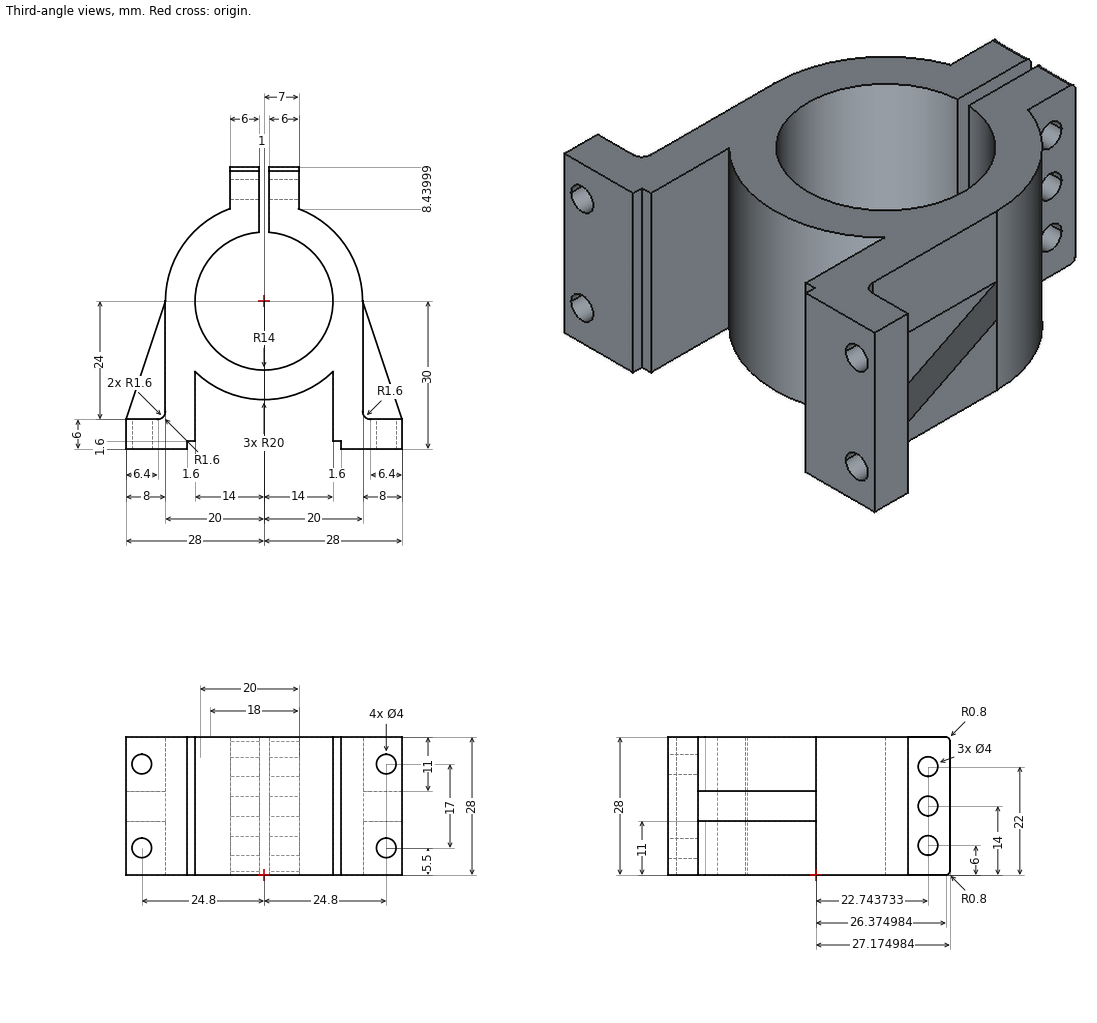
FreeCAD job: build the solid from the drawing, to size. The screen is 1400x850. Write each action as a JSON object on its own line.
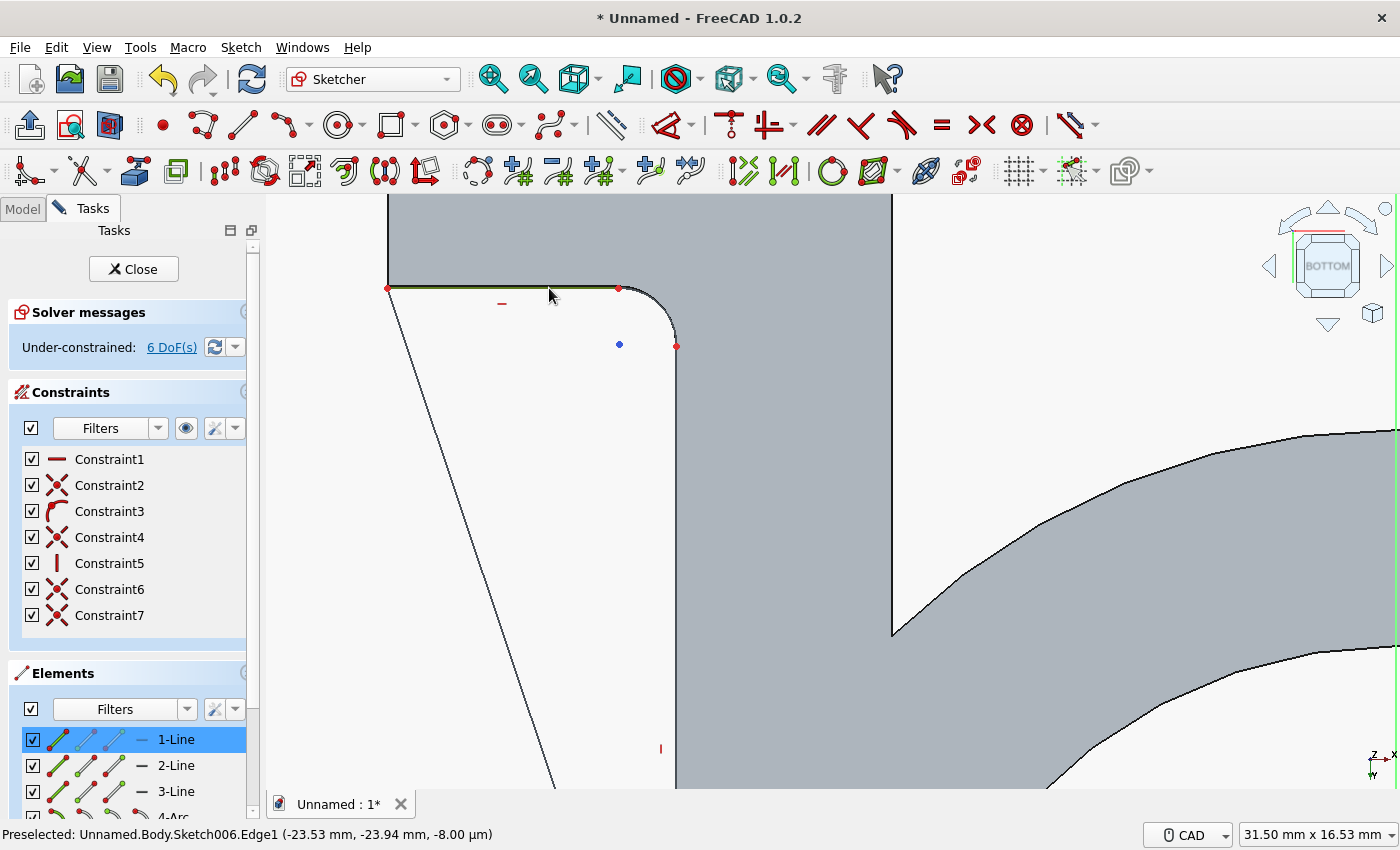
{"action": "left_click", "coordinate": [670, 320]}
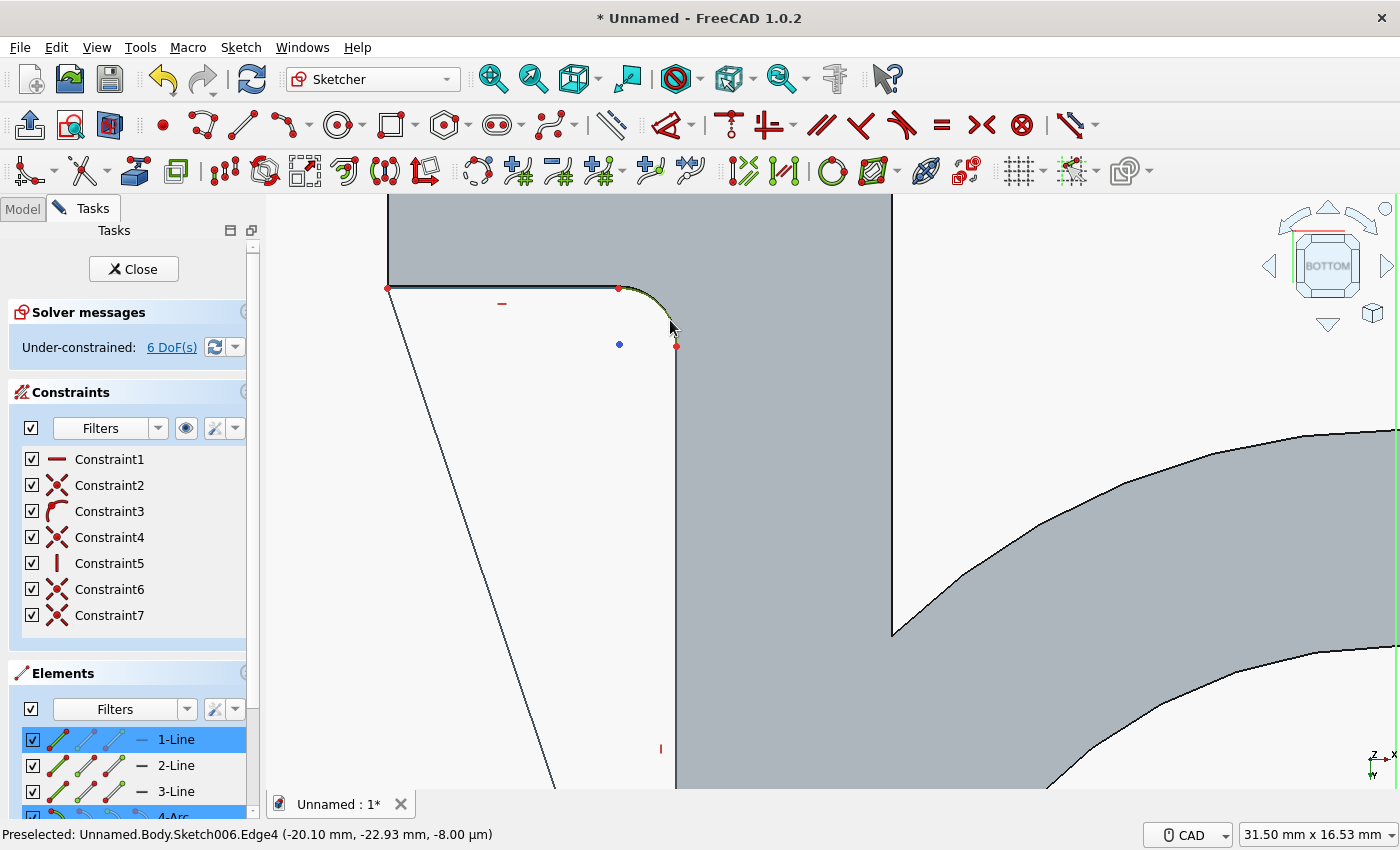
{"action": "left_click", "coordinate": [902, 126]}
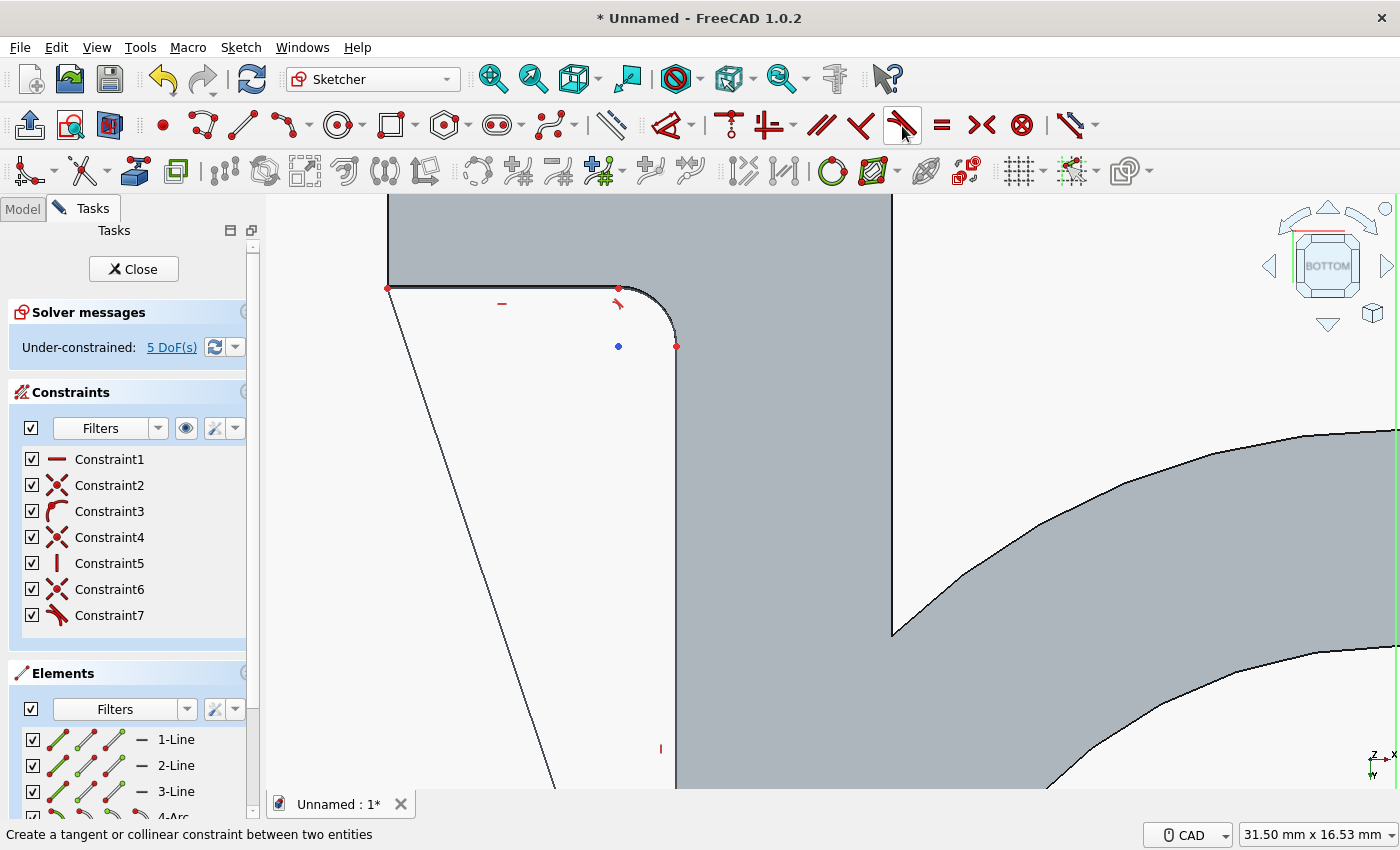
{"action": "left_click", "coordinate": [676, 587]}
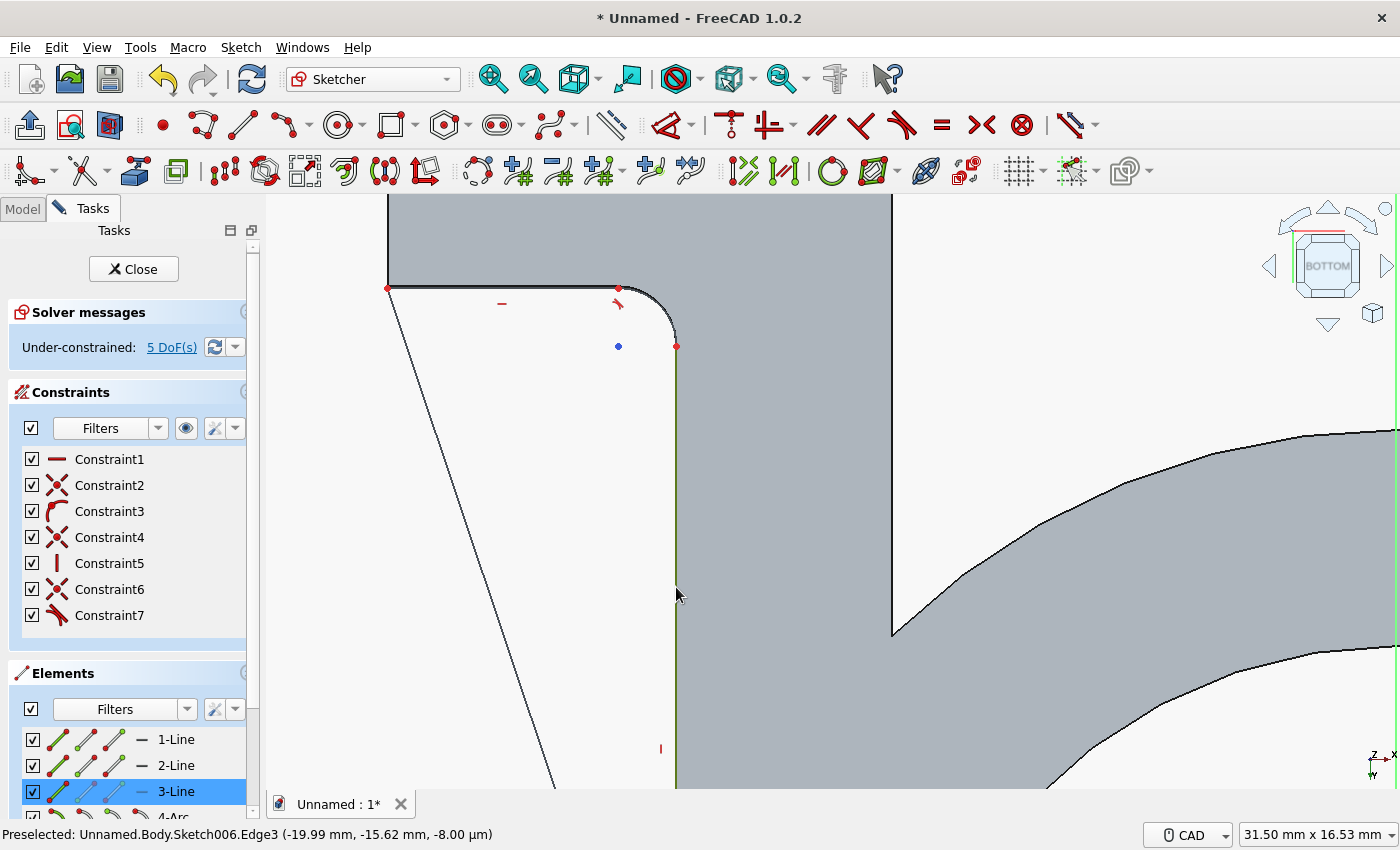
{"action": "left_click", "coordinate": [670, 320]}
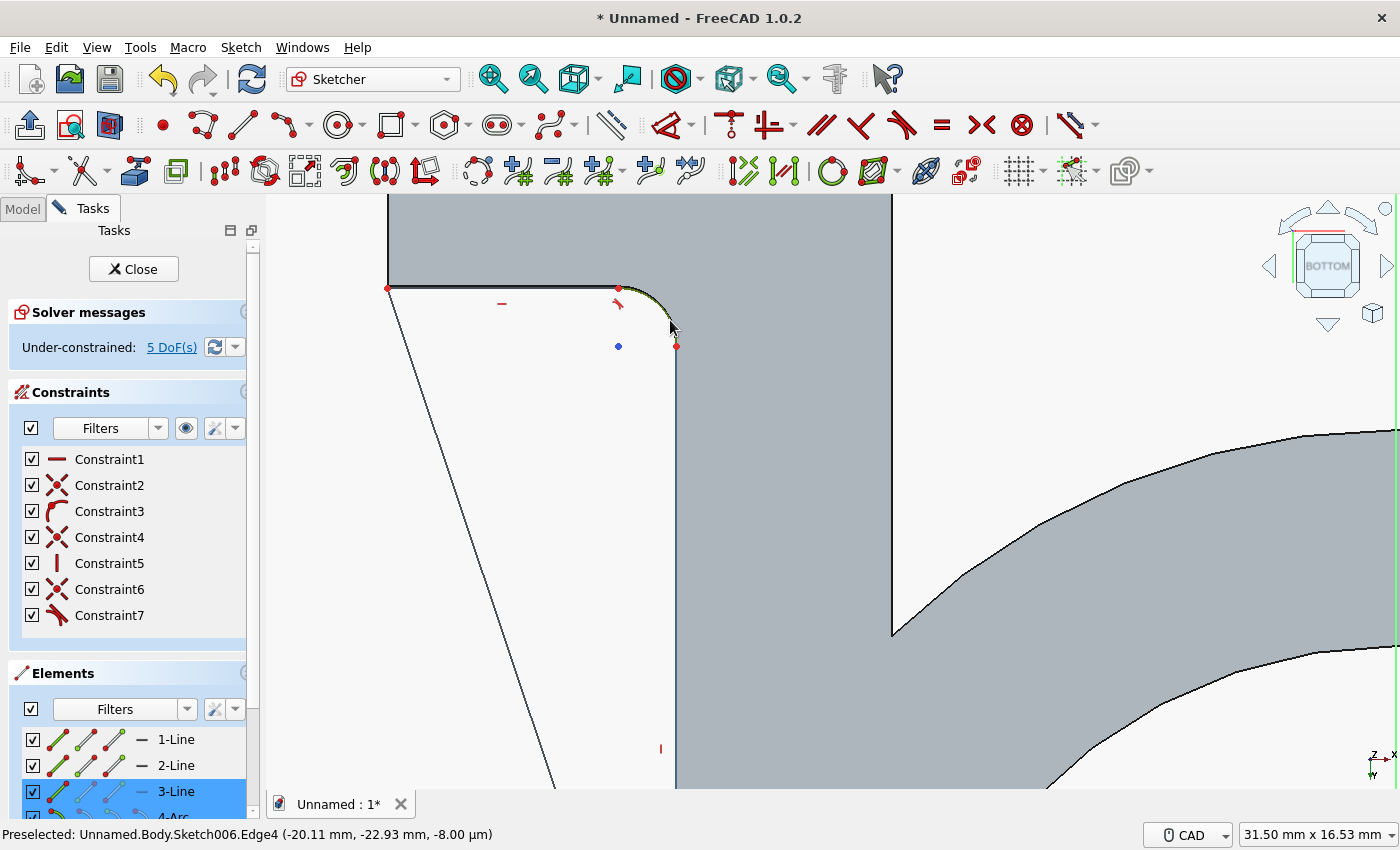
{"action": "left_click", "coordinate": [902, 126]}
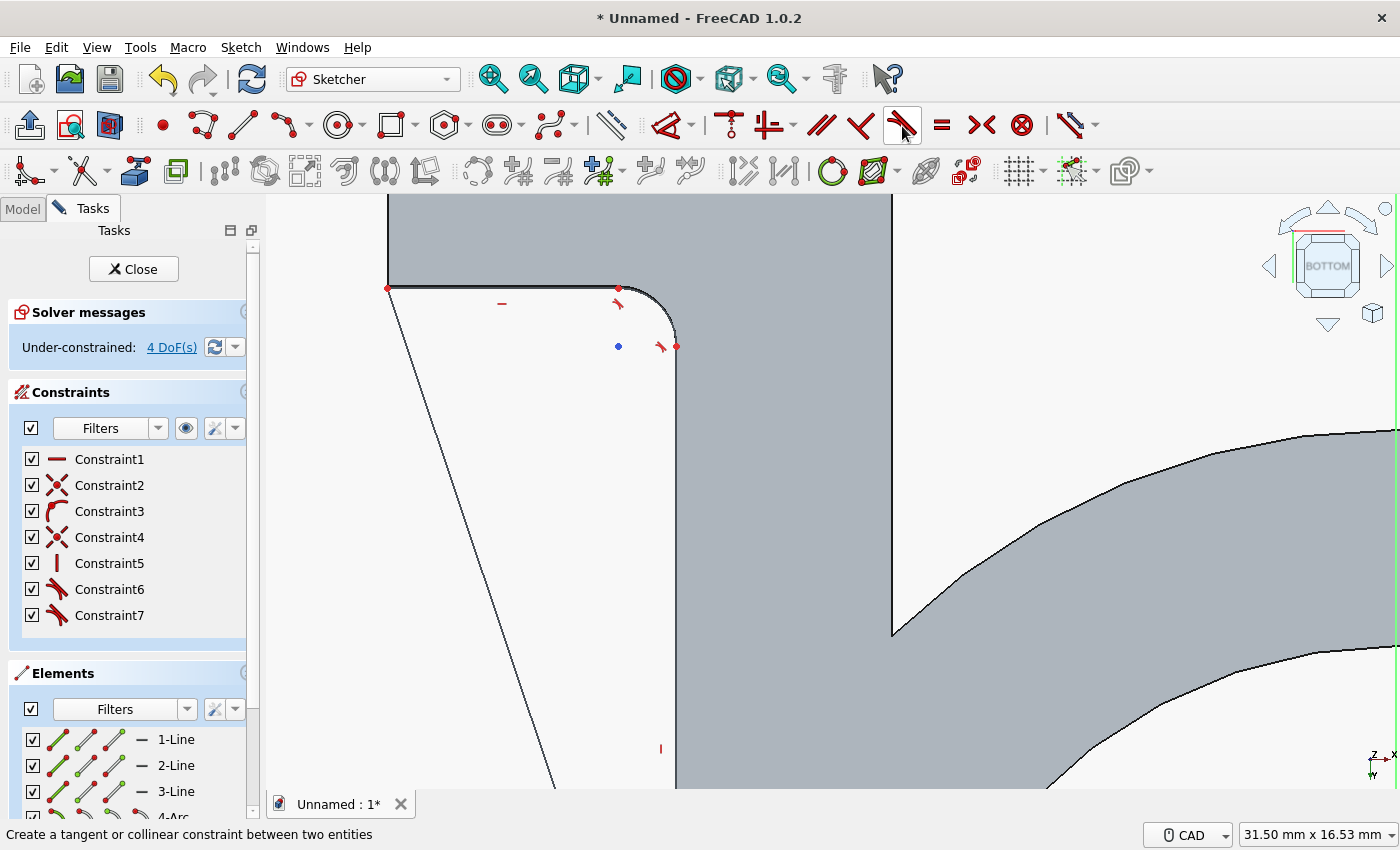
{"action": "left_click", "coordinate": [666, 126]}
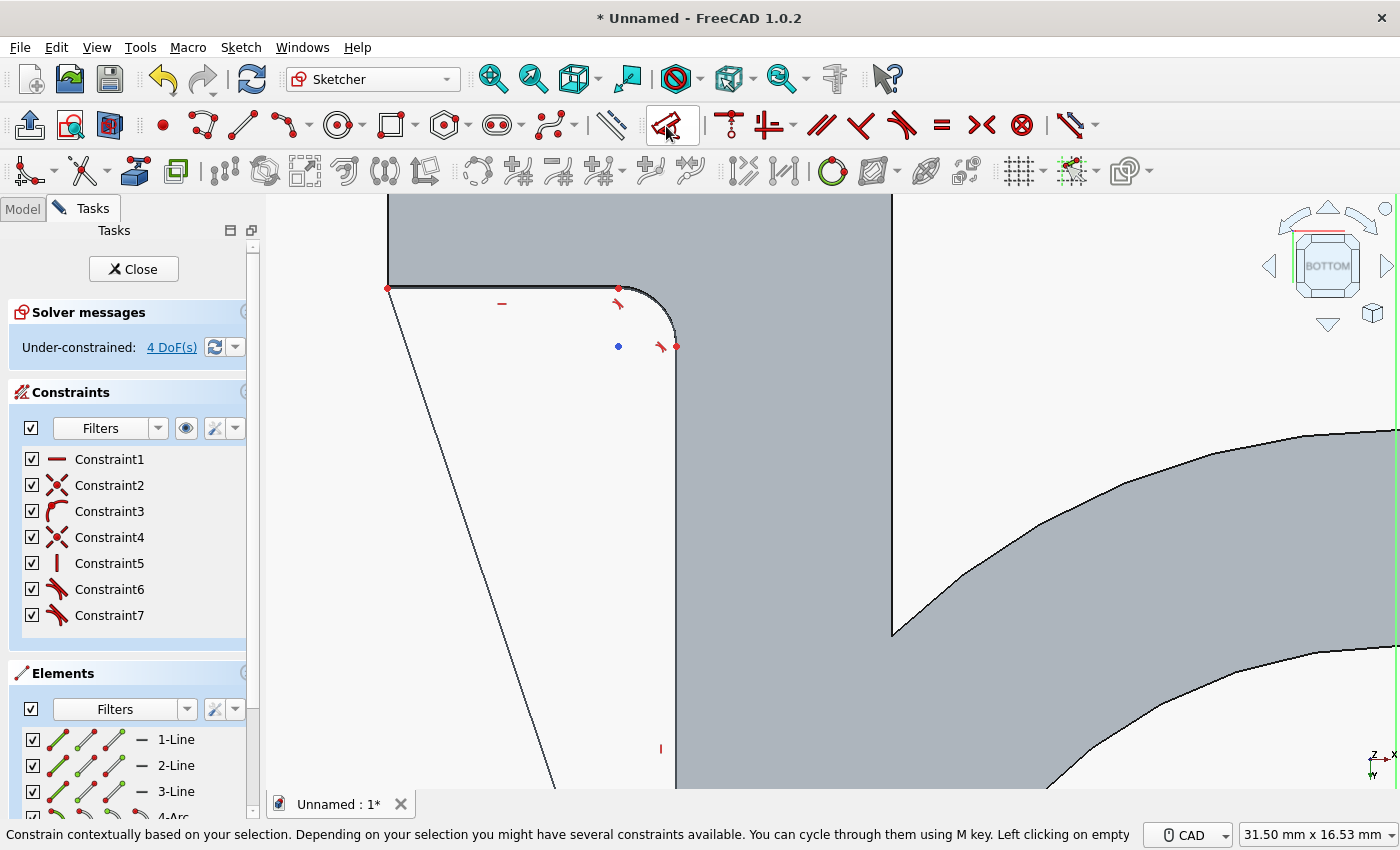
{"action": "left_click", "coordinate": [670, 320]}
{"action": "left_click", "coordinate": [699, 306]}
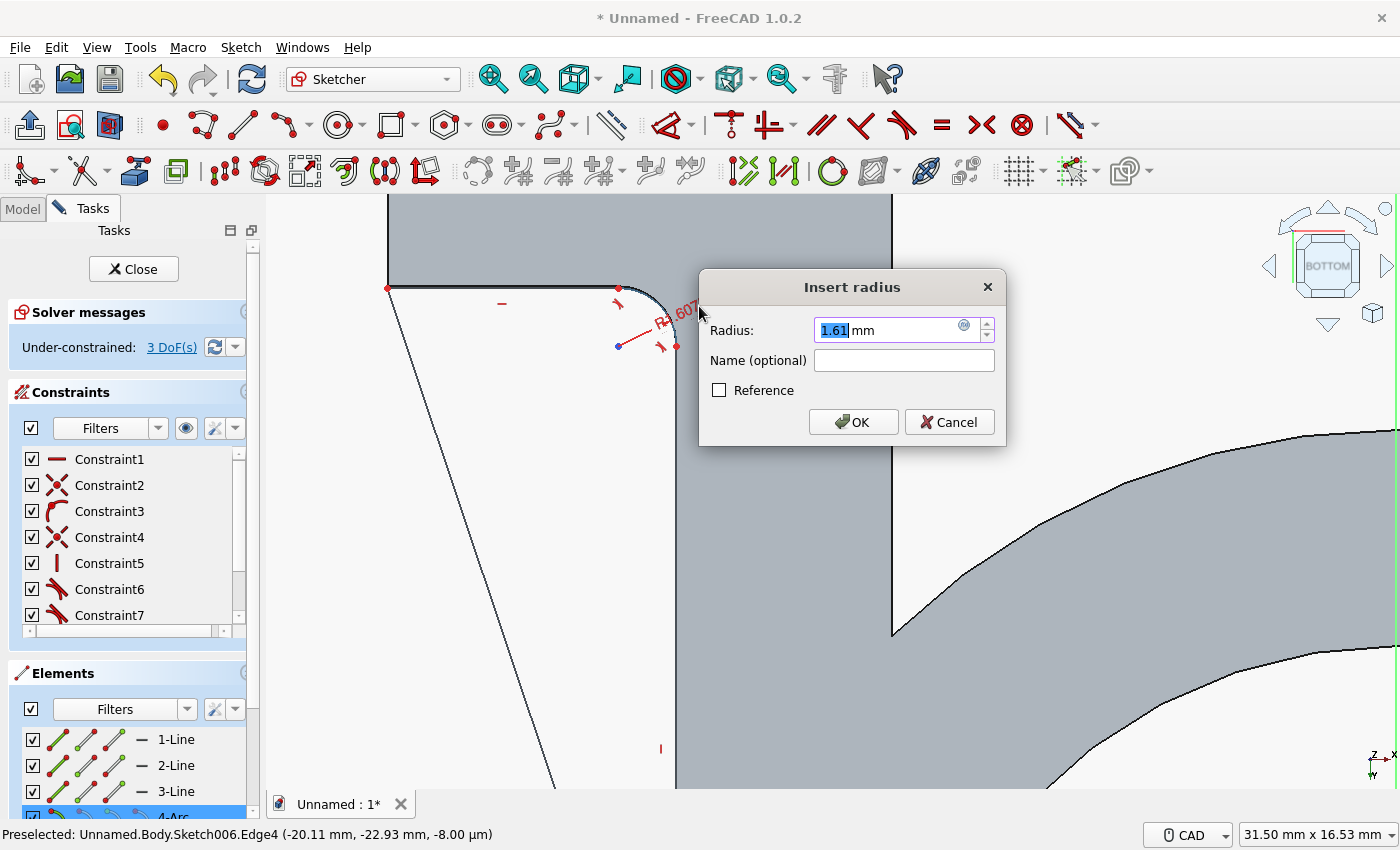
{"action": "type", "text": "1.6"}
{"action": "key", "text": "Return"}